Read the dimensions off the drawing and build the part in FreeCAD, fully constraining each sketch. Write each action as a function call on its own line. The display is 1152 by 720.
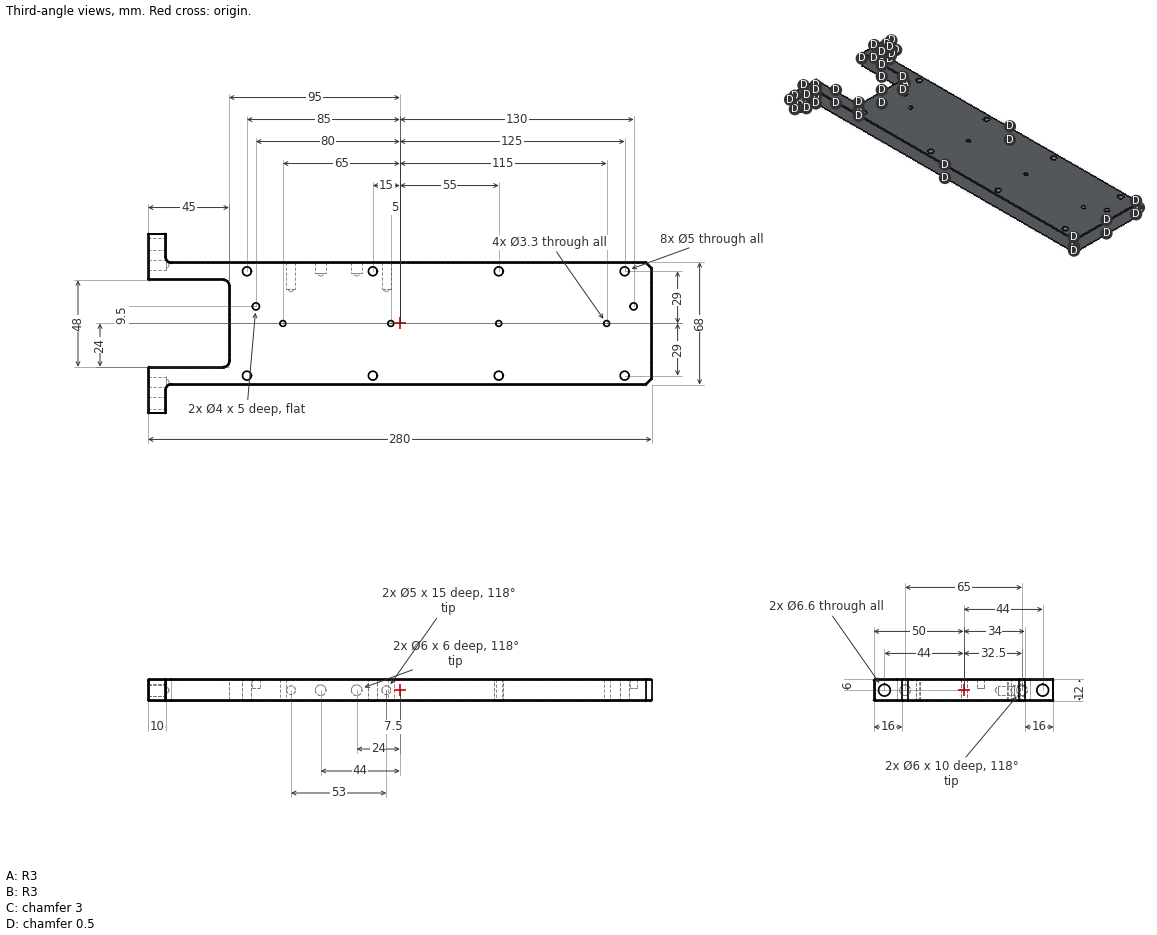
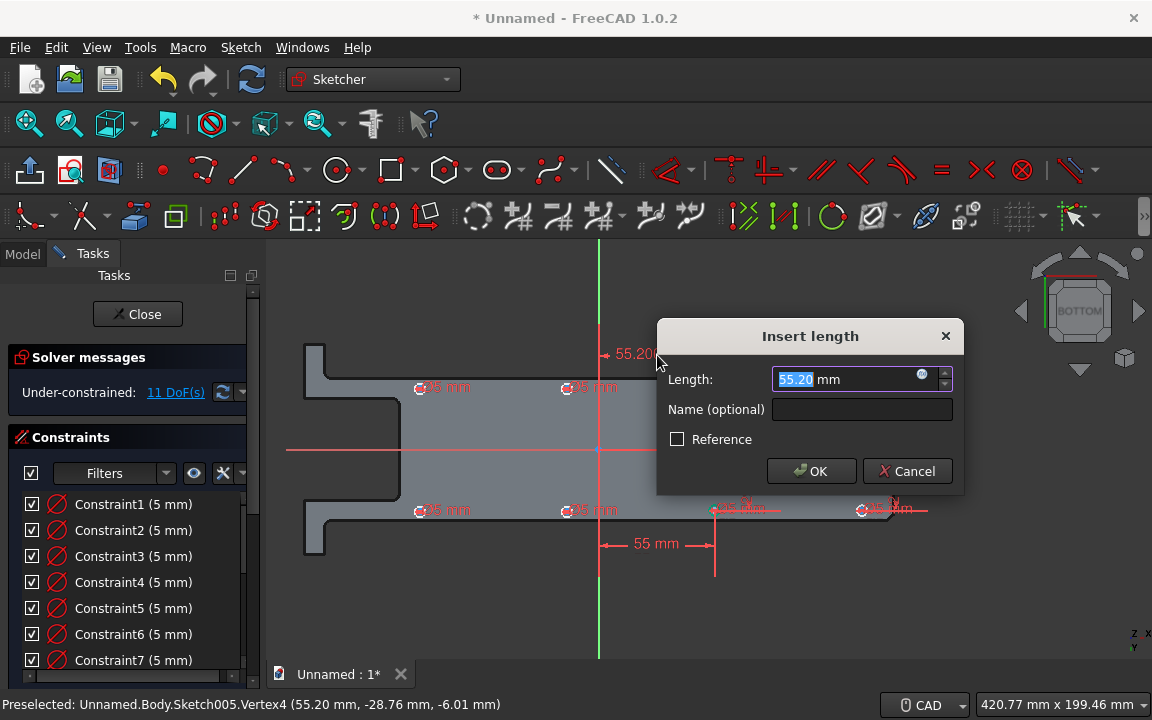
text(55)
key(Return)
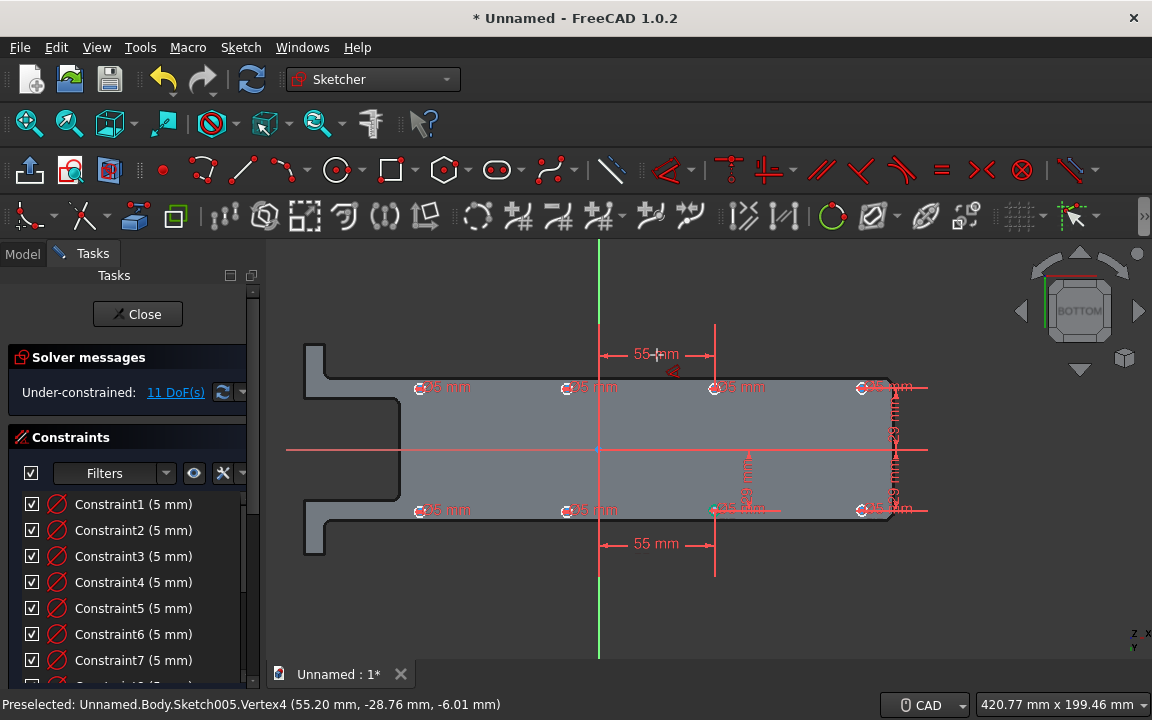
click(715, 389)
click(749, 419)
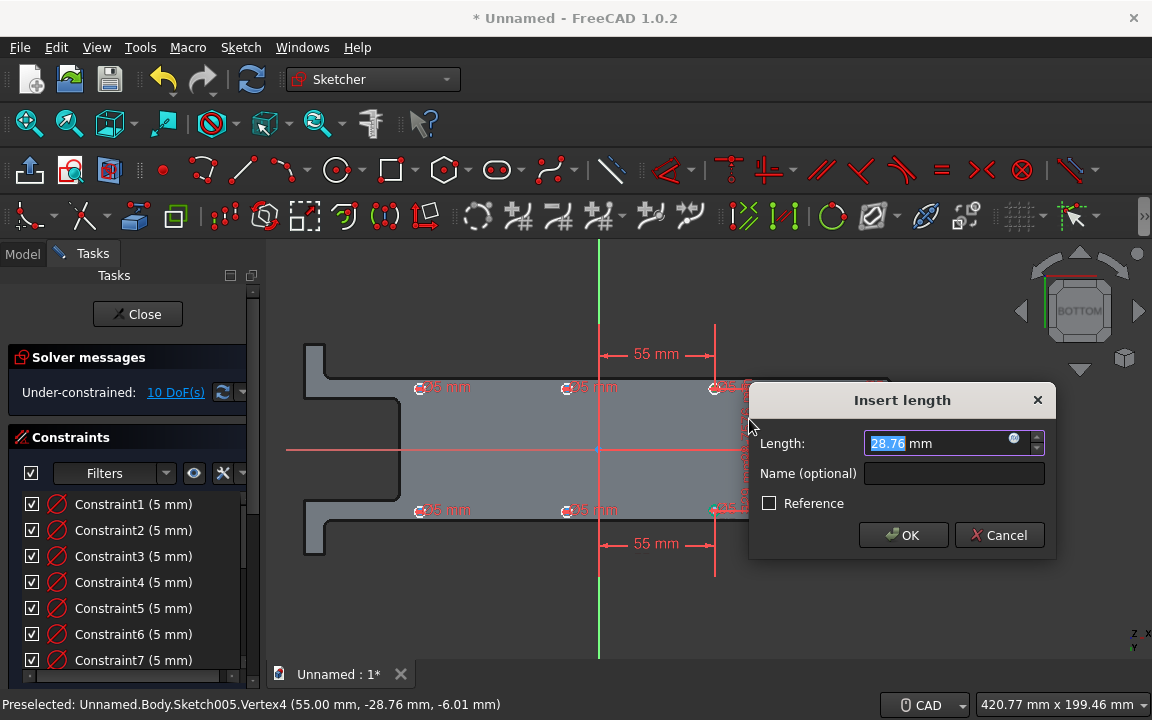
text(29)
key(Return)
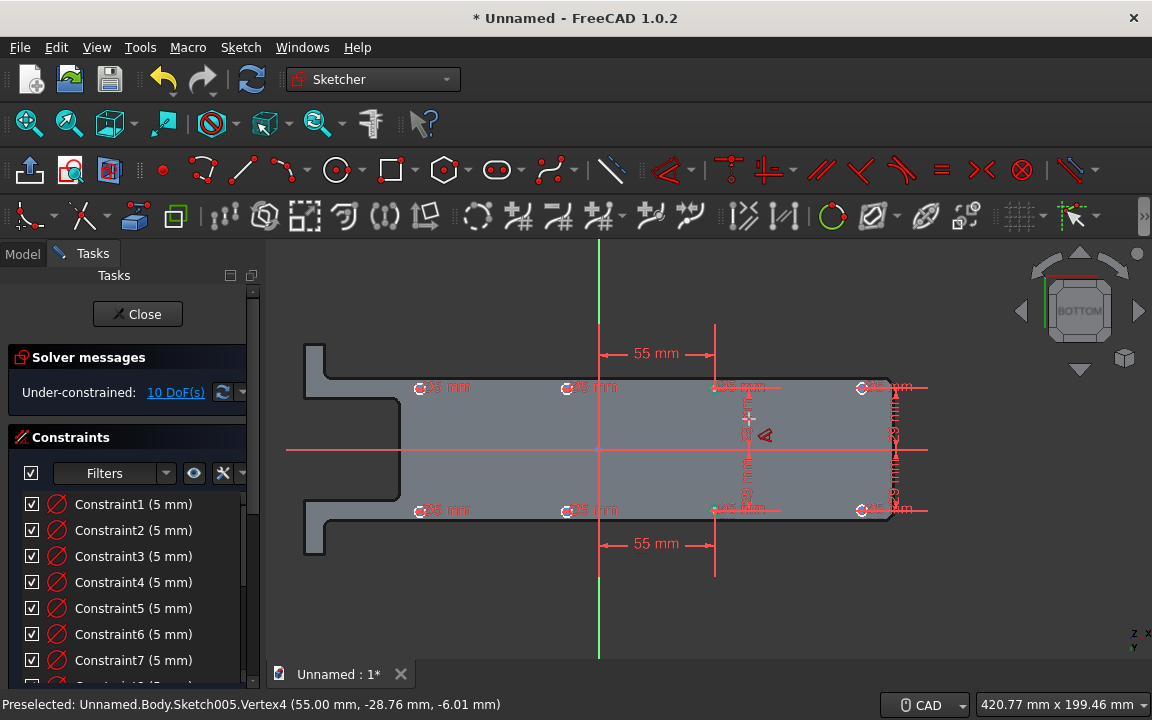
scroll(567, 512, up, 2)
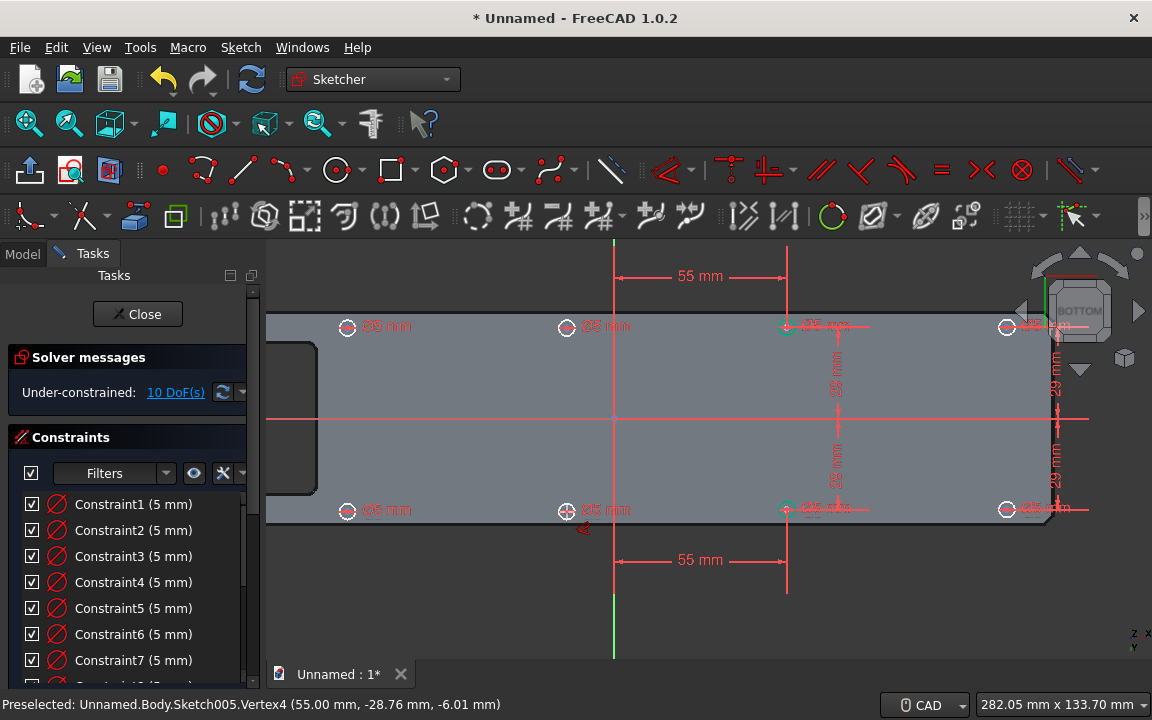
click(567, 512)
click(591, 546)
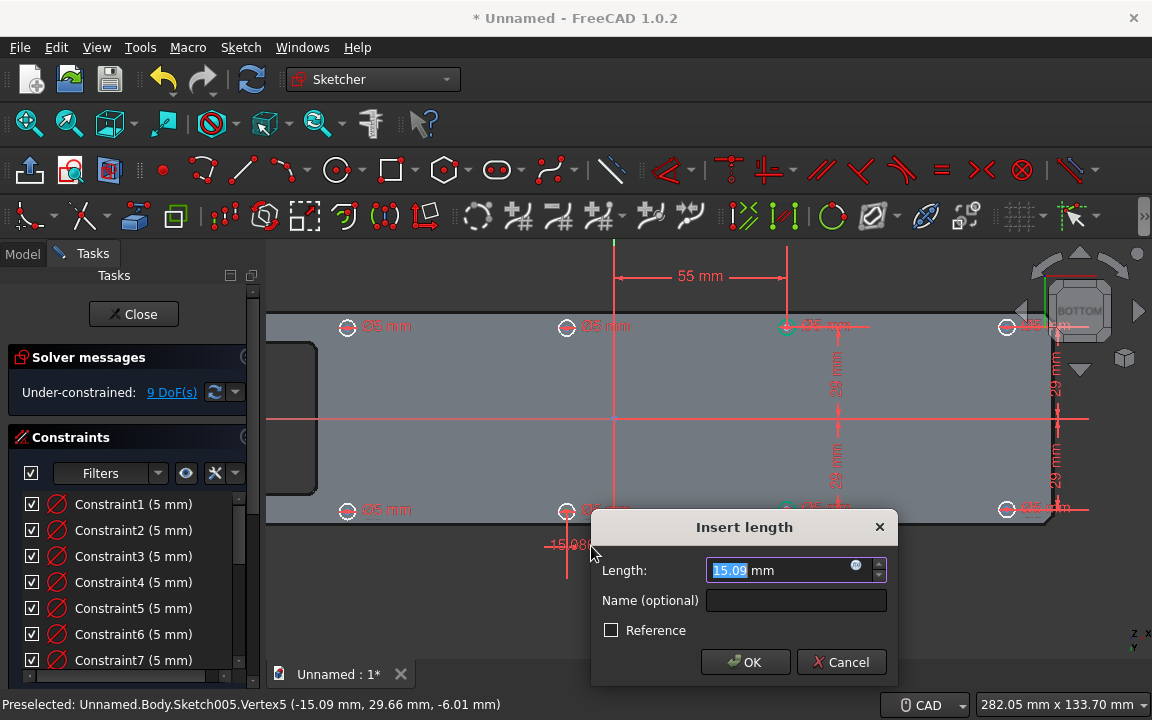
text(15)
key(Return)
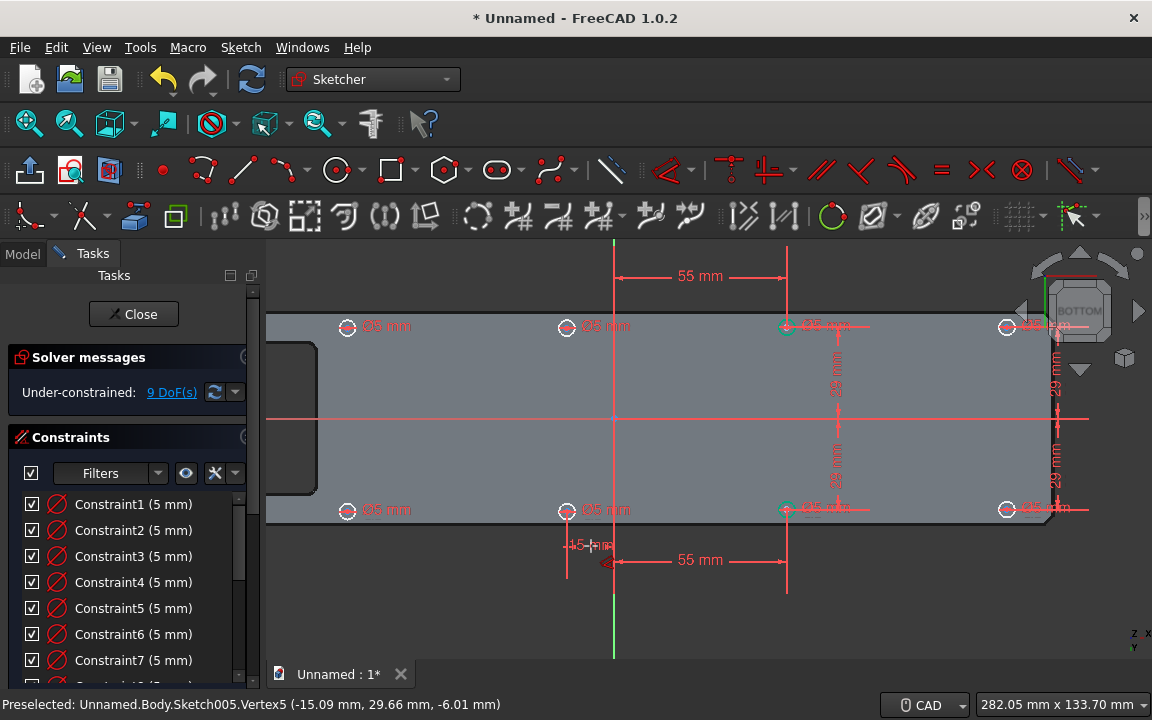
click(567, 512)
click(533, 465)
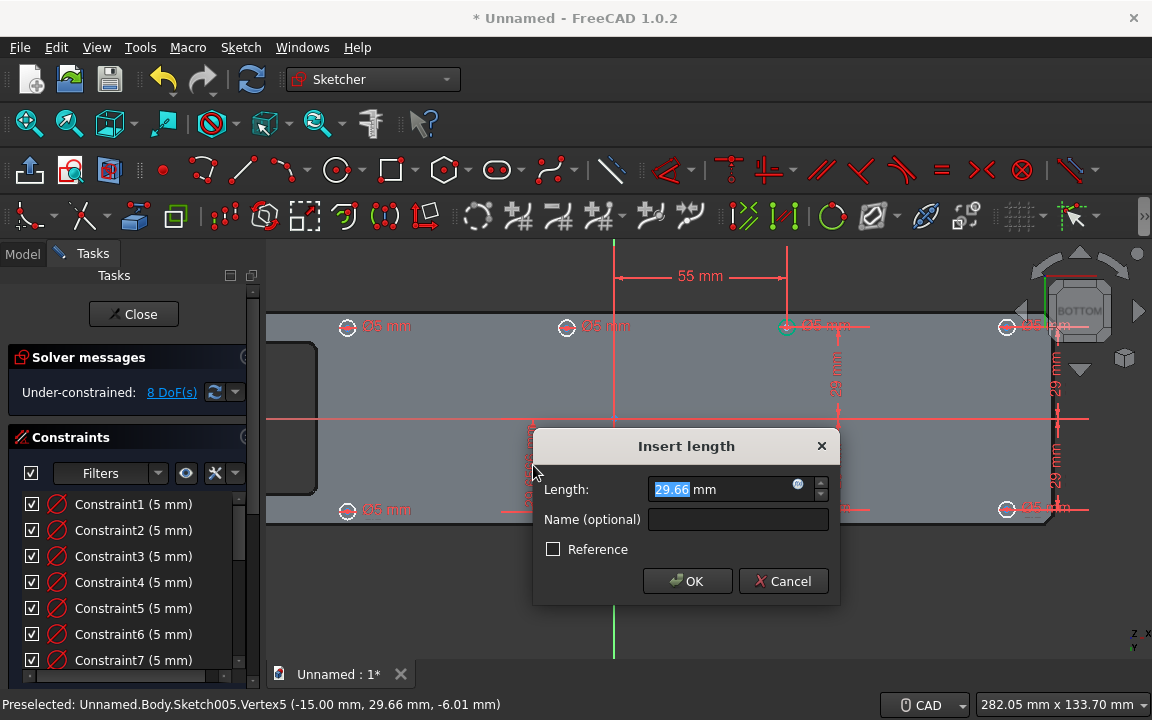
text(29)
key(Return)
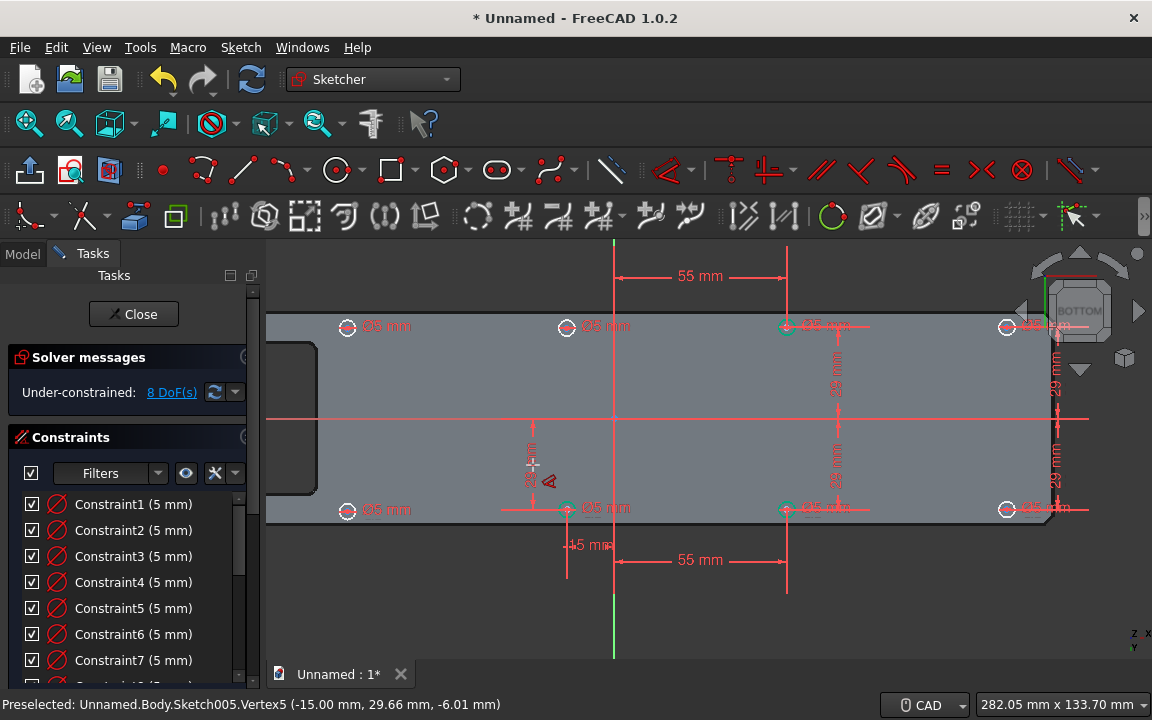
click(567, 328)
click(591, 294)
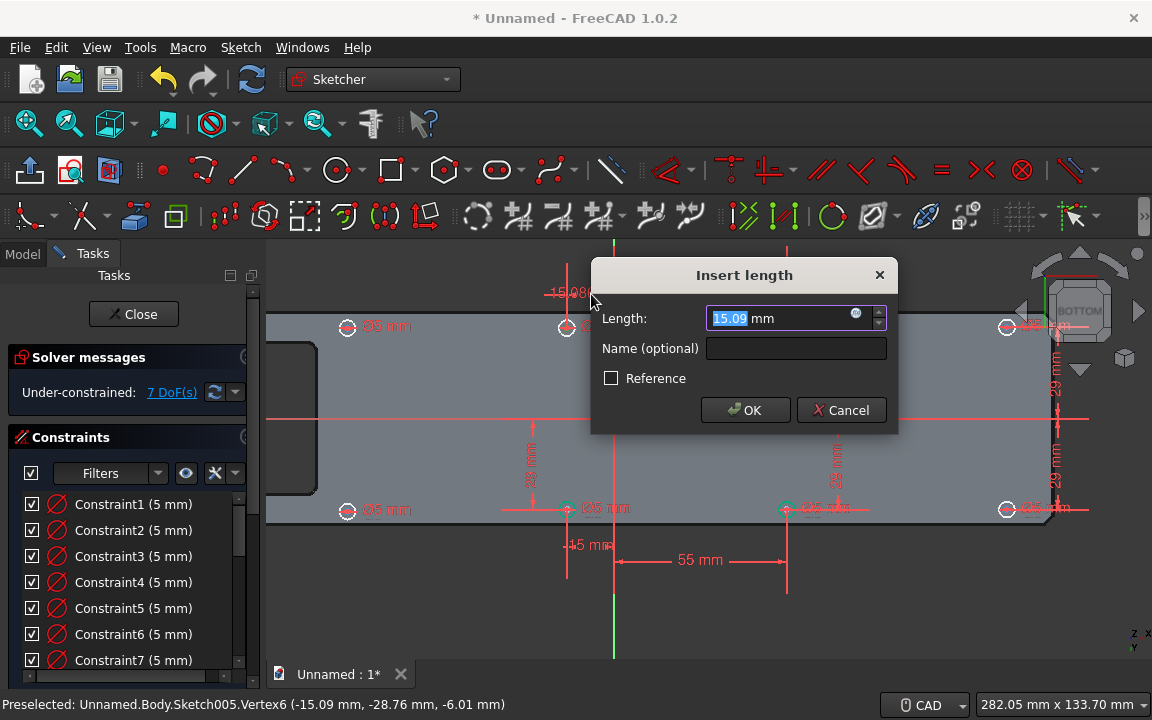
text(15)
key(Return)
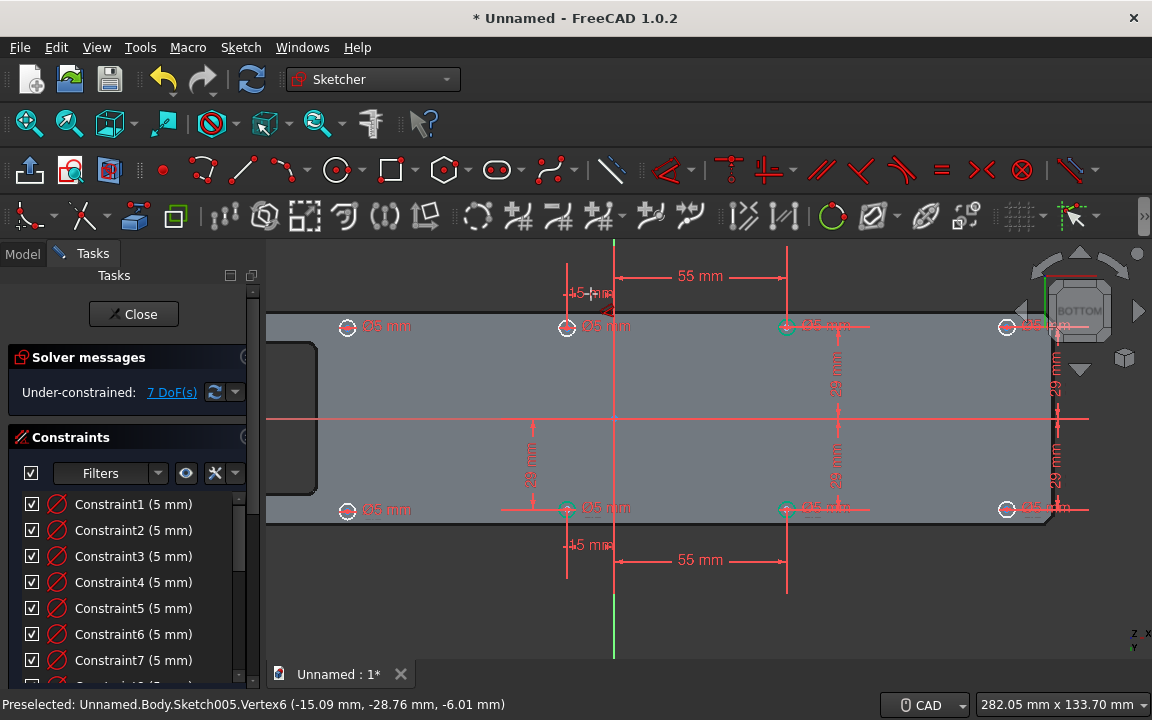
click(567, 328)
click(533, 373)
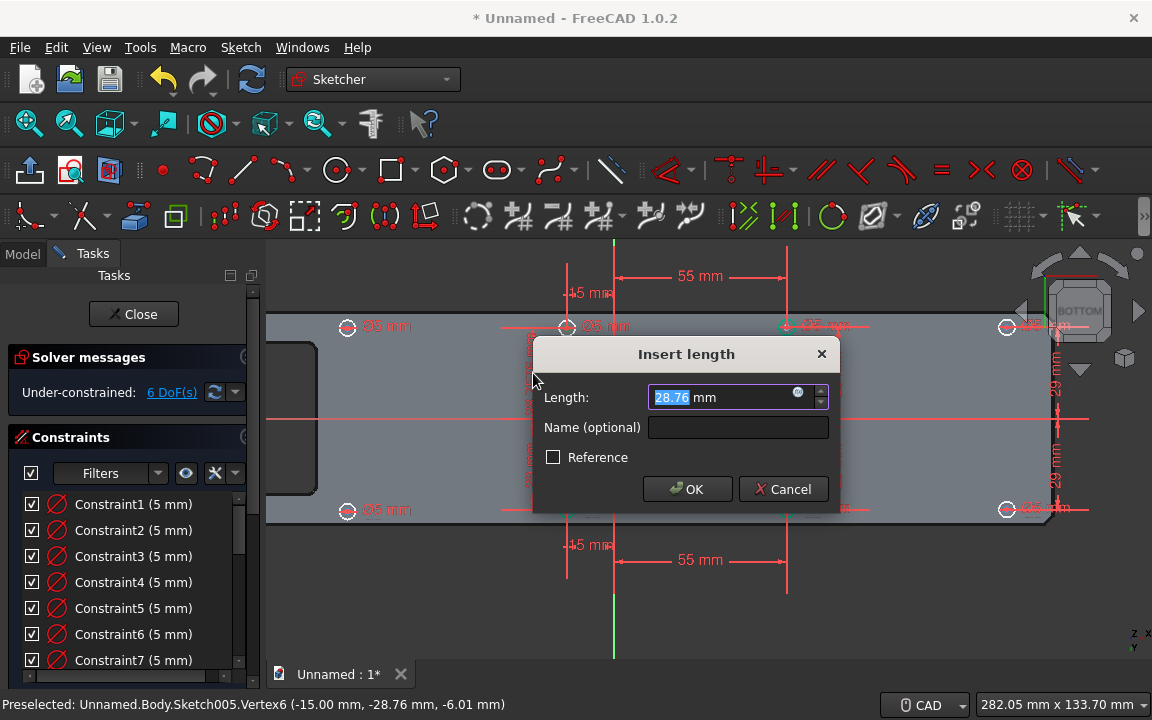
text(29)
key(Return)